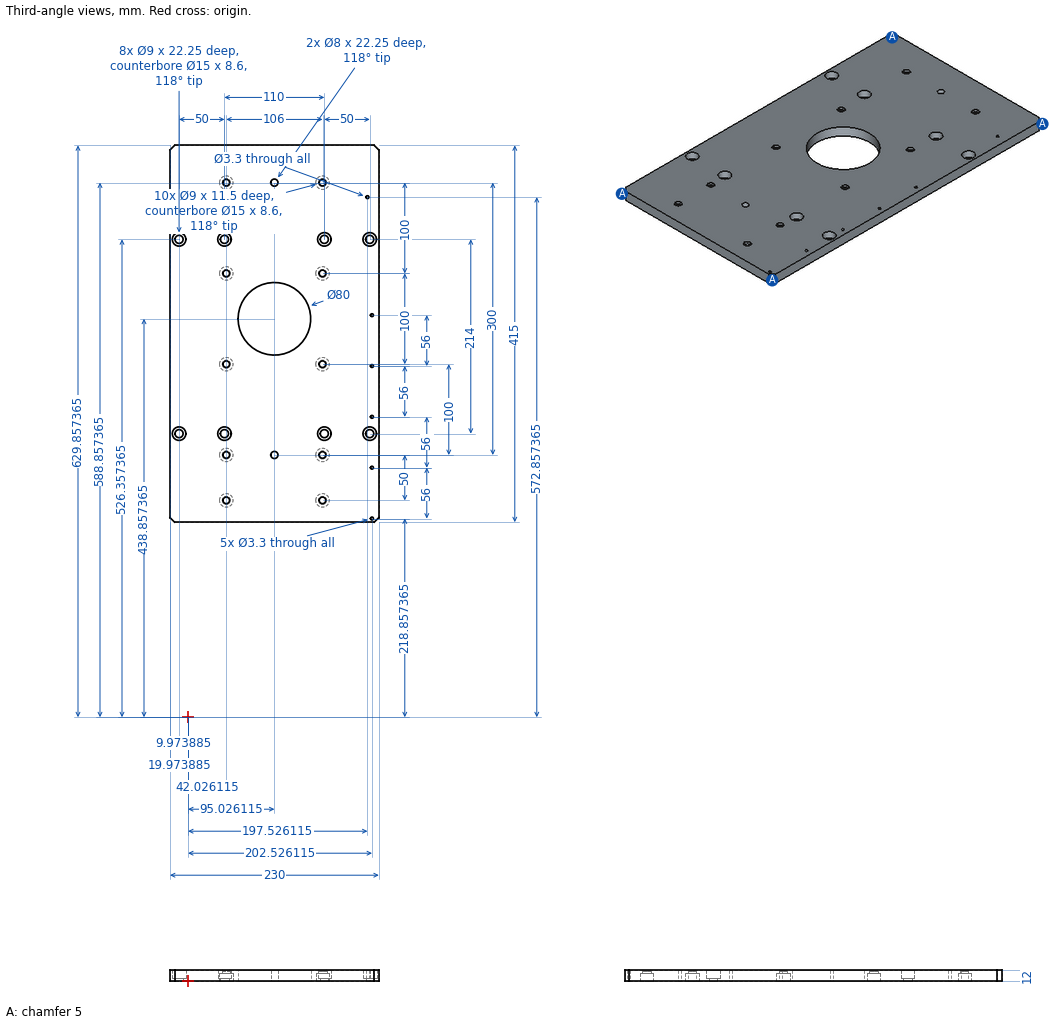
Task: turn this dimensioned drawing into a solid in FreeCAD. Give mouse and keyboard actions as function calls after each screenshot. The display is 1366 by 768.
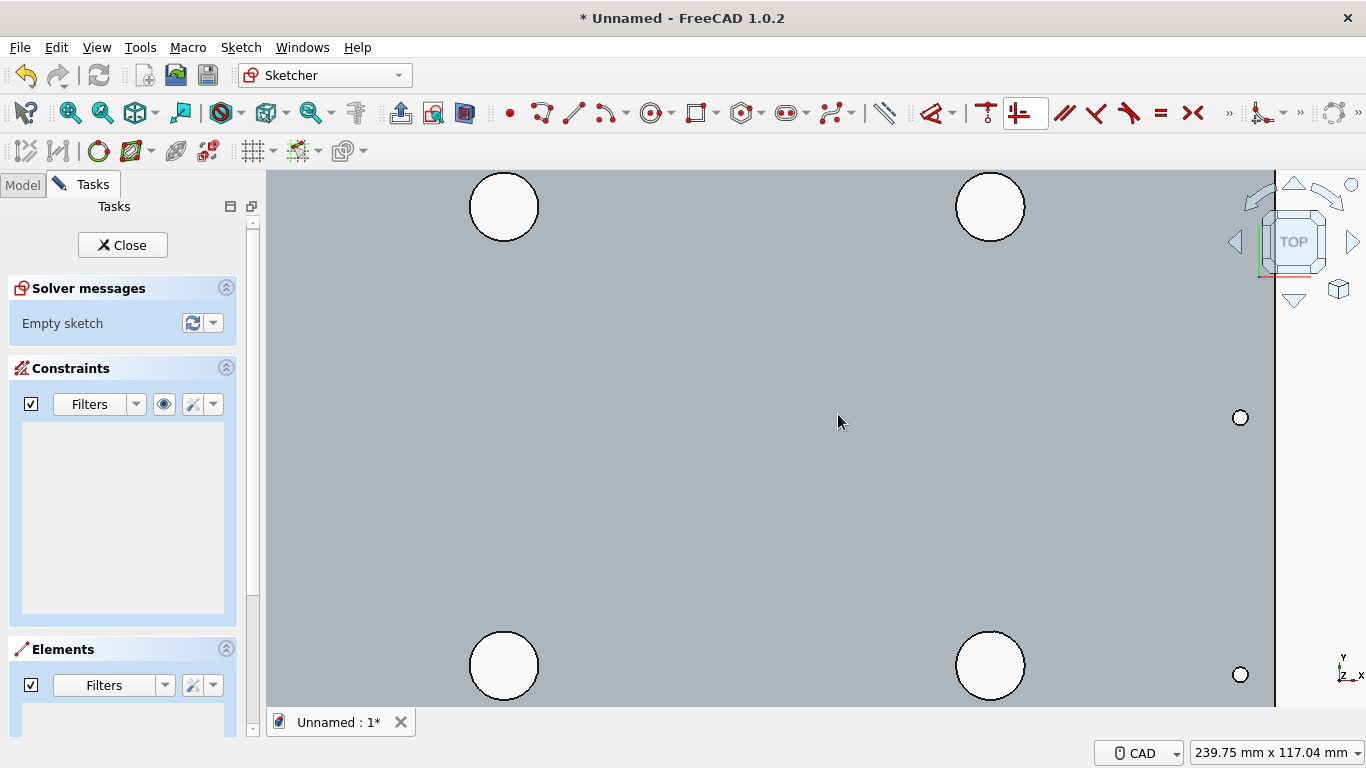
click(652, 114)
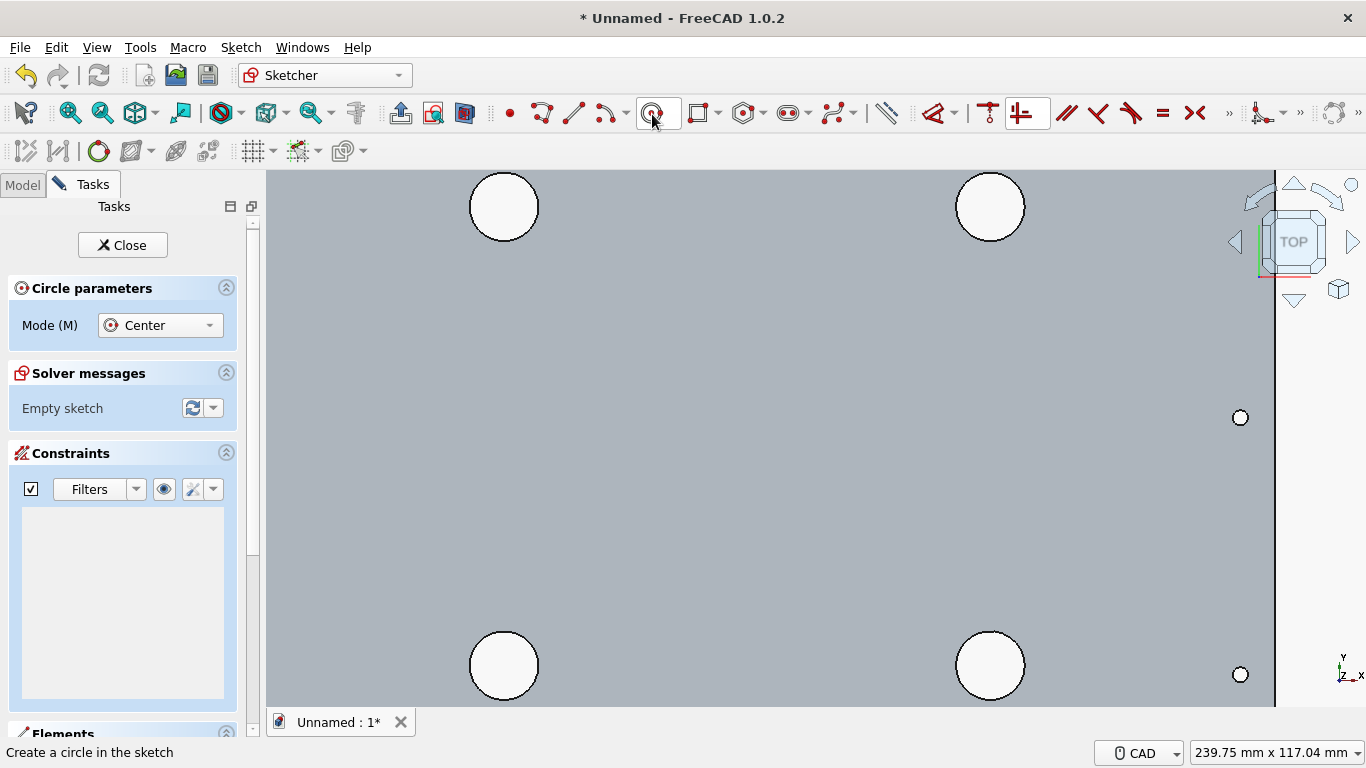
click(747, 436)
move(877, 306)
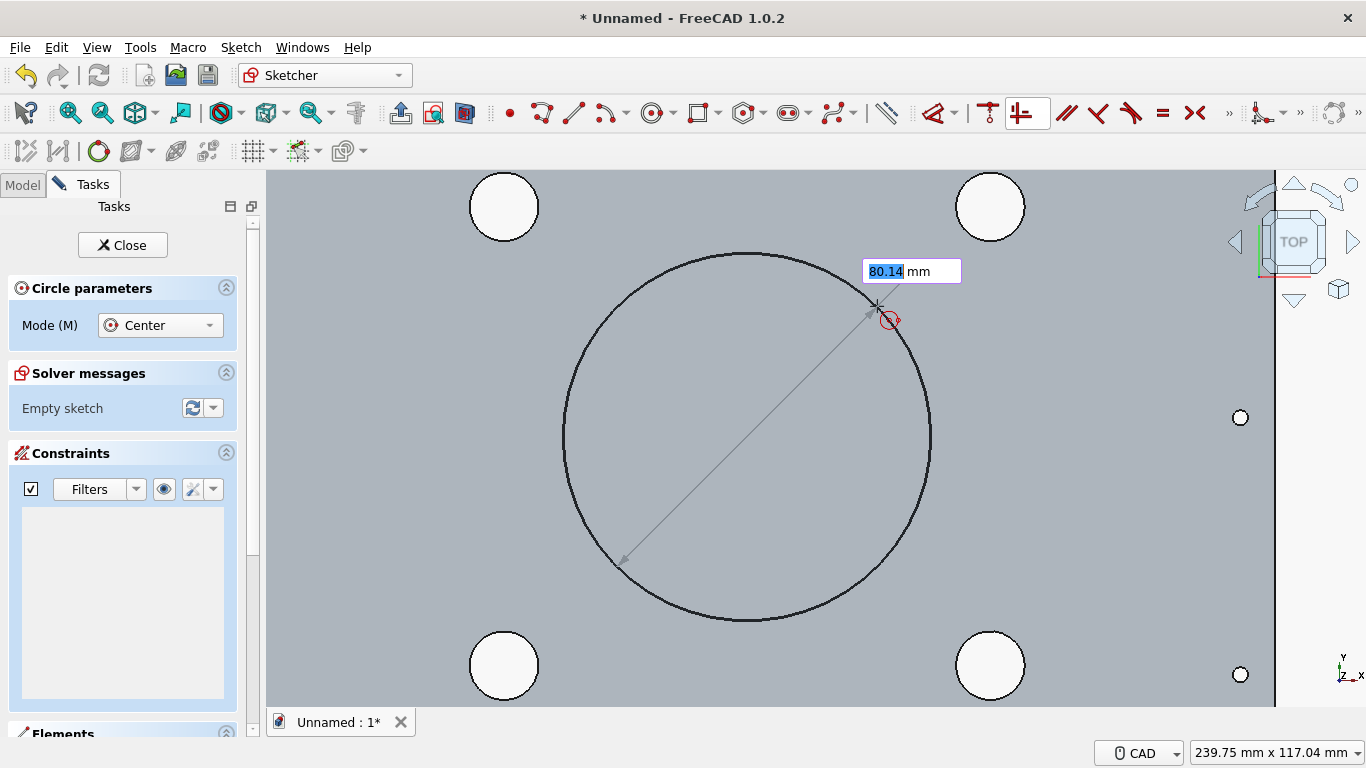
text(80)
key(Return)
key(Escape)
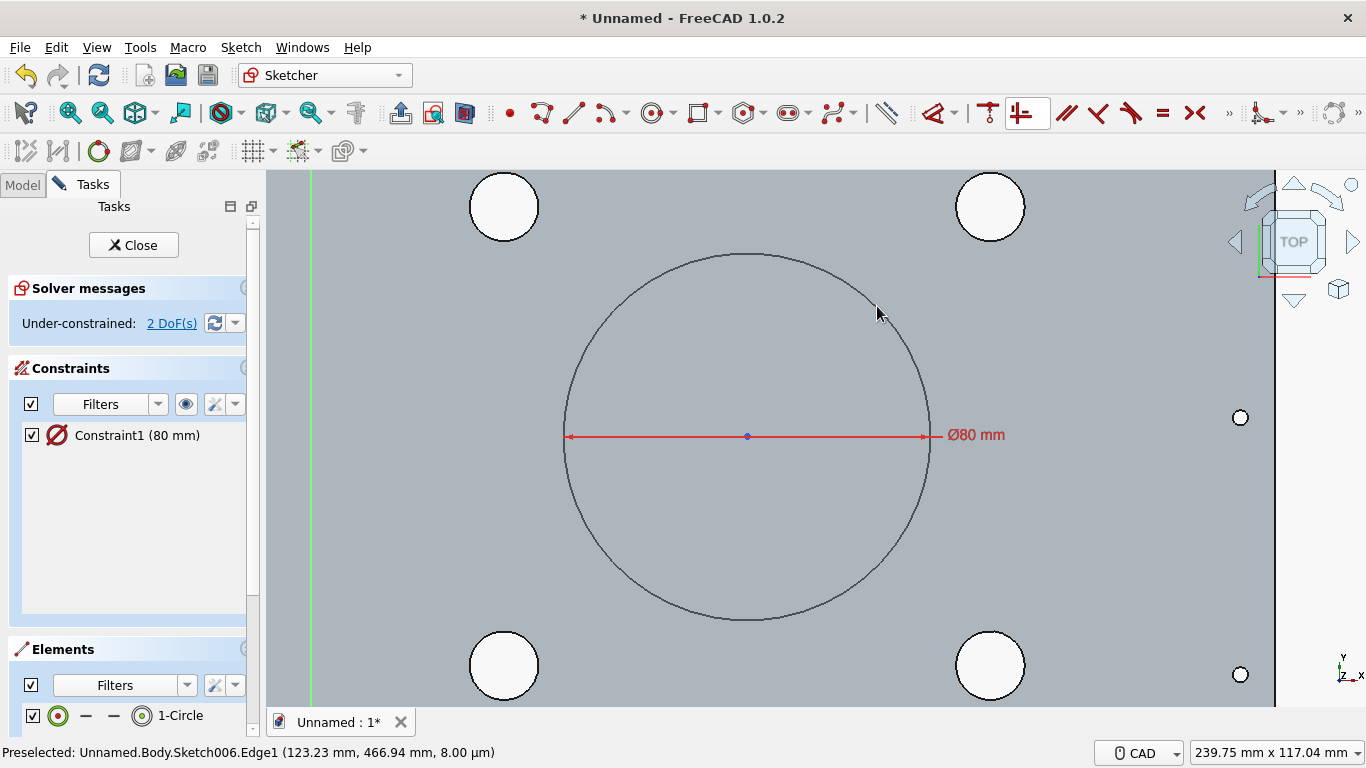
click(934, 114)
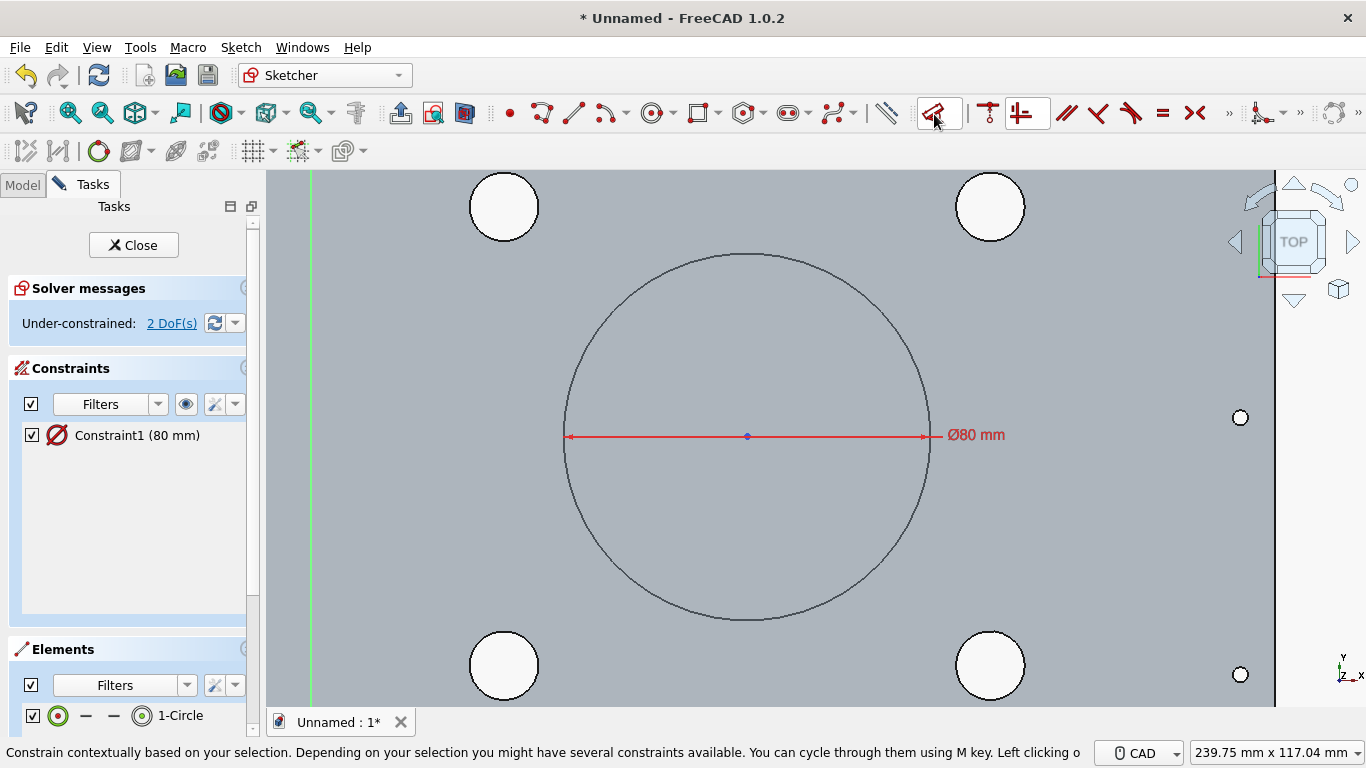
click(747, 437)
click(529, 403)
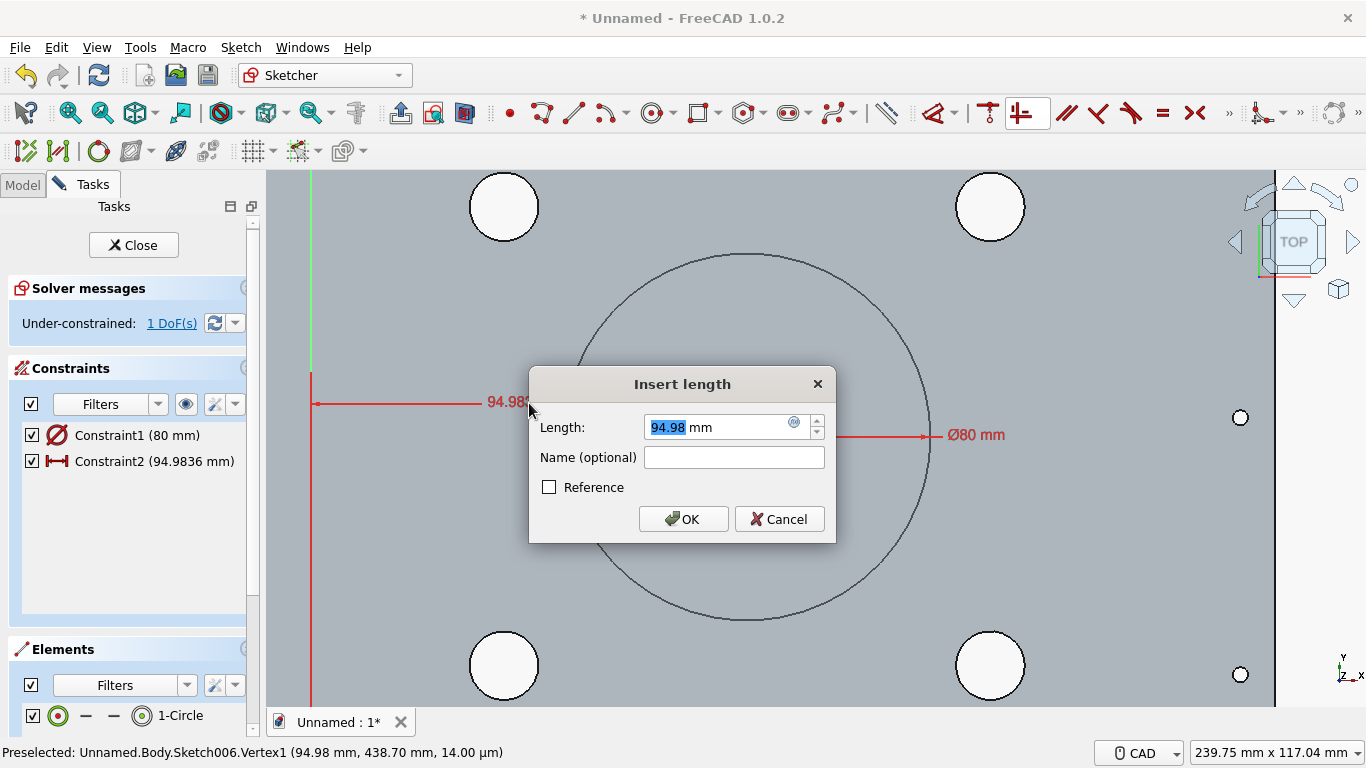
text(95.026115)
key(Return)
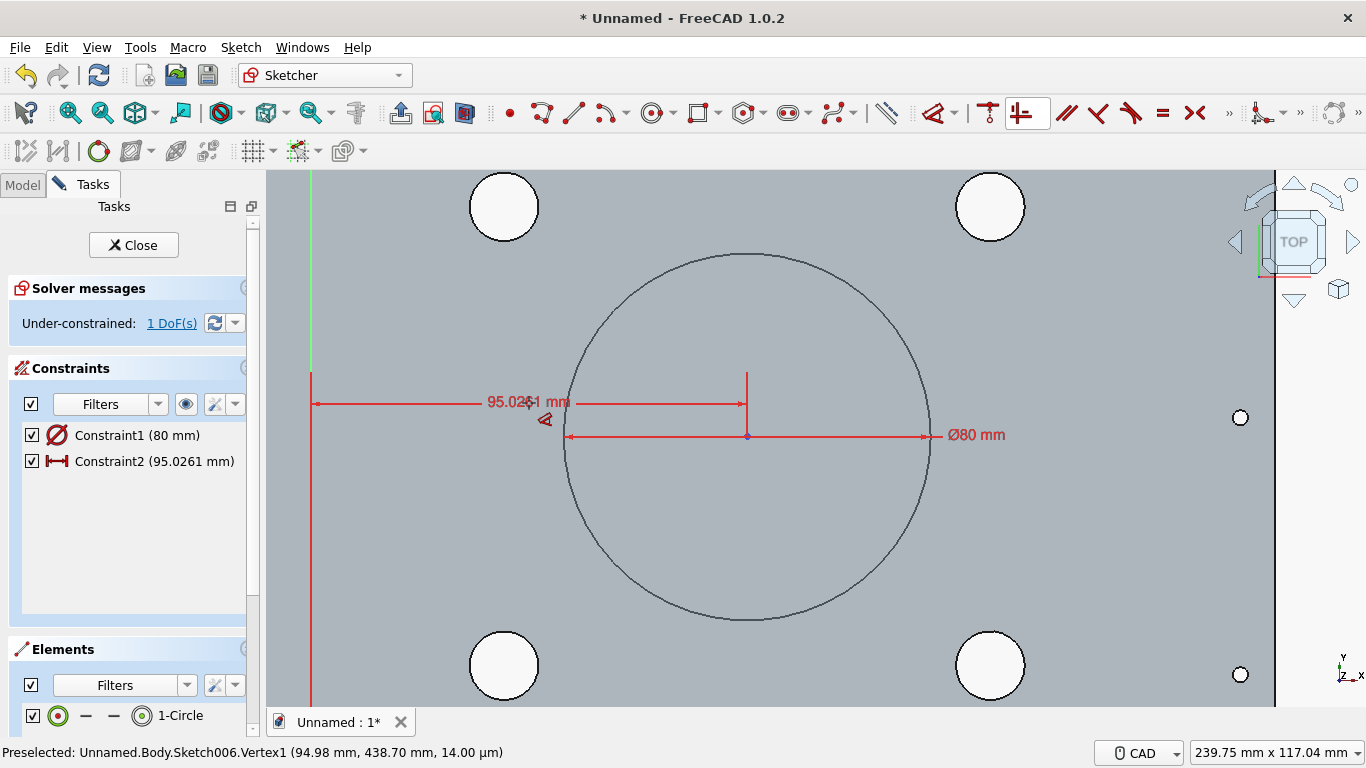
click(747, 437)
click(781, 558)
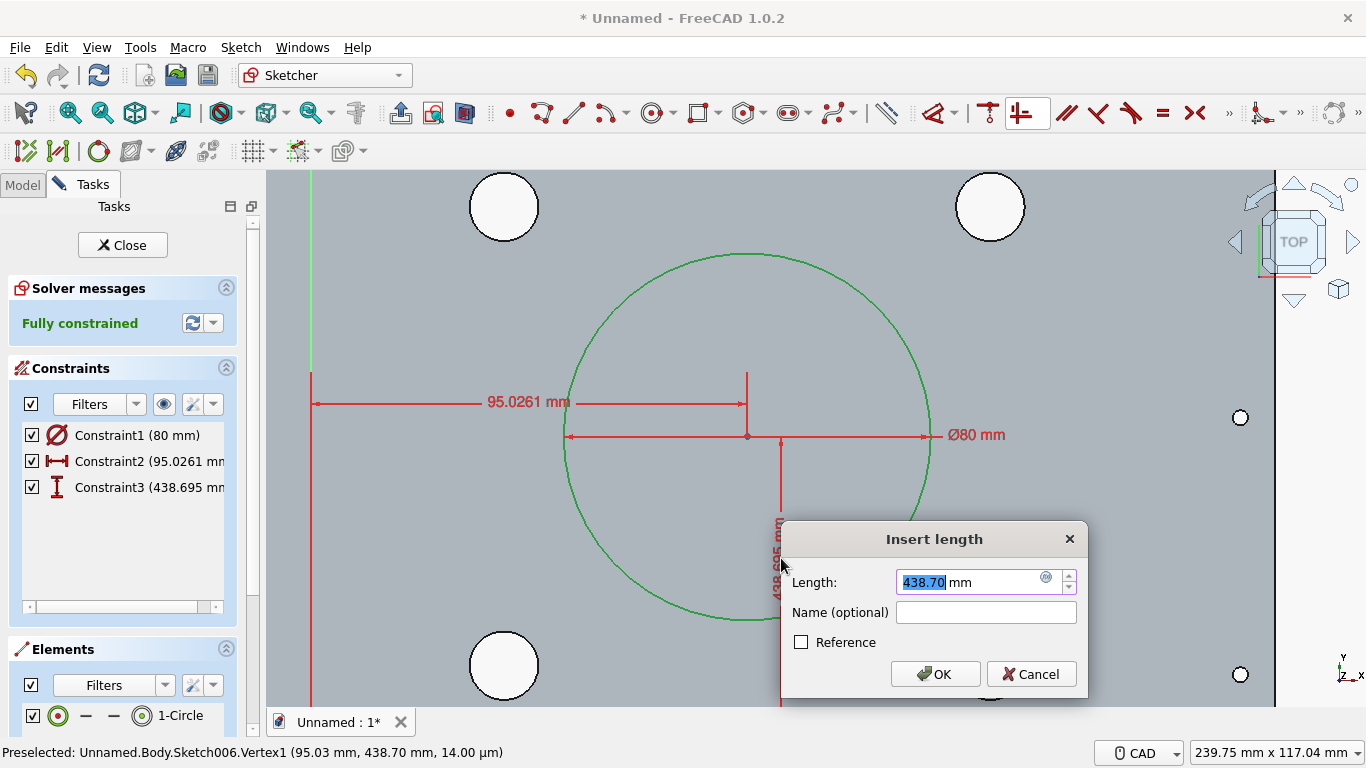
text(438.857365)
key(Return)
key(Escape)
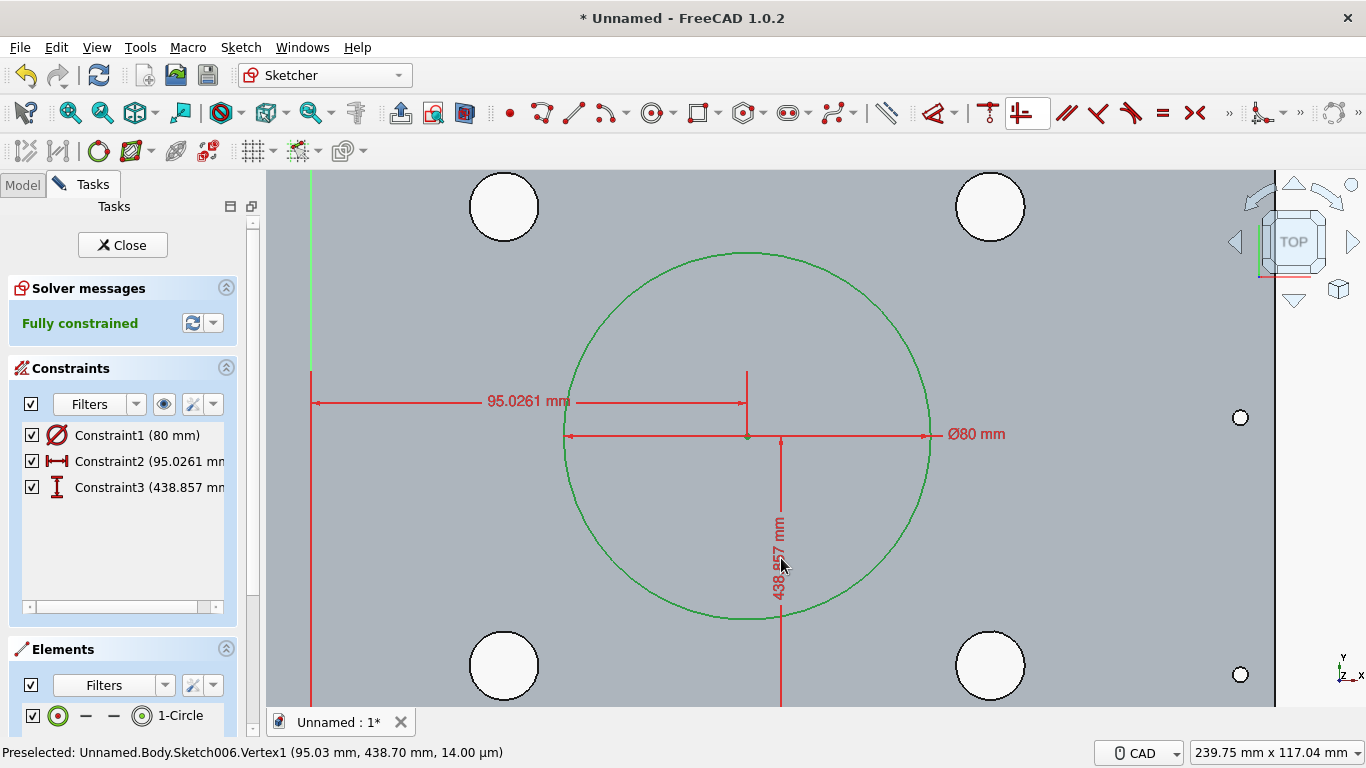
click(123, 245)